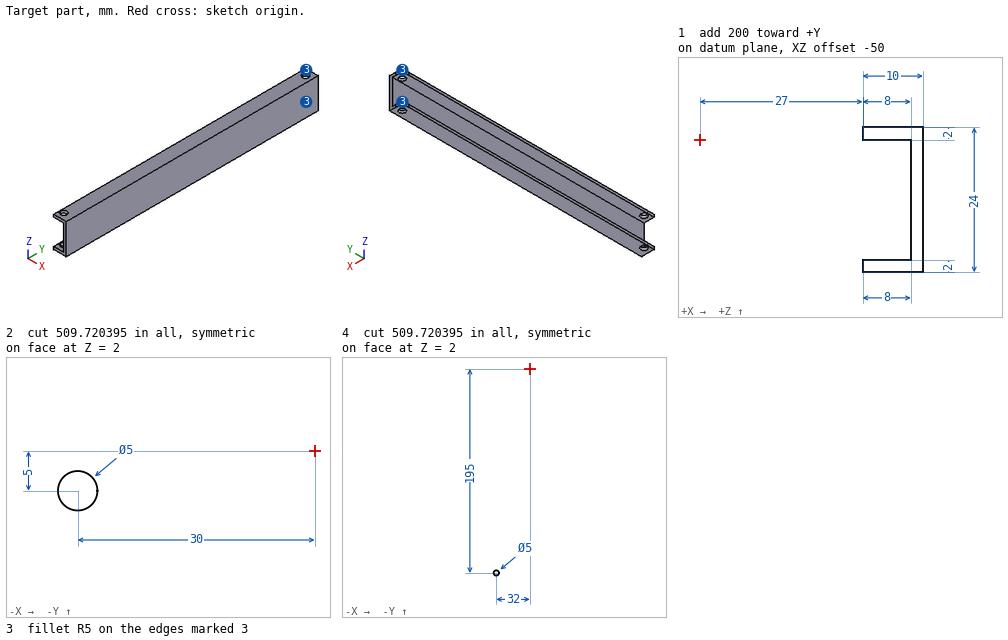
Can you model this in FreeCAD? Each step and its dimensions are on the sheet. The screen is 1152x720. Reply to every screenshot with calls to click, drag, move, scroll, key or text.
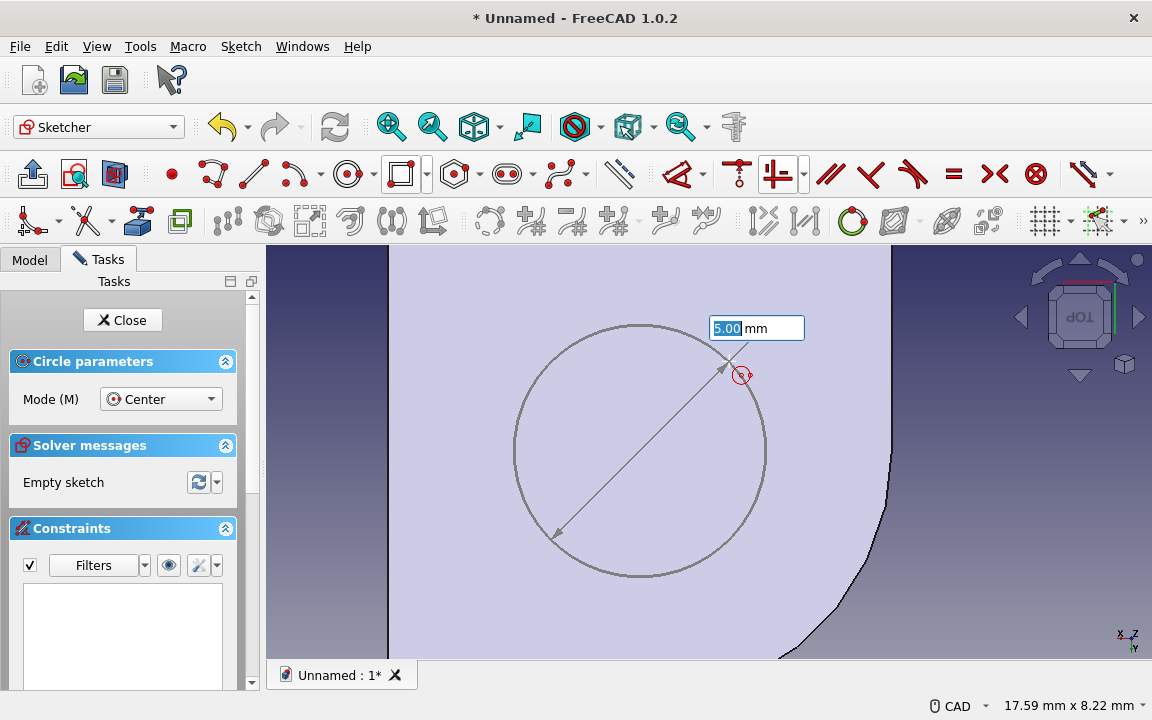
text(5)
key(Return)
key(Escape)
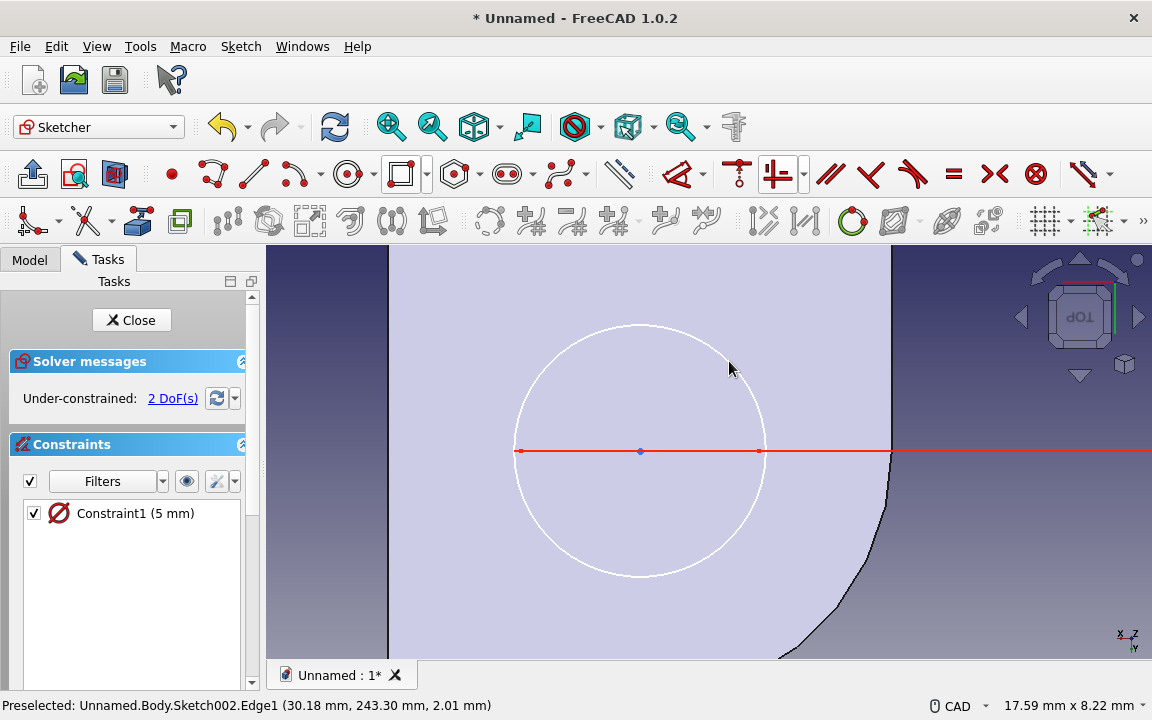
click(676, 174)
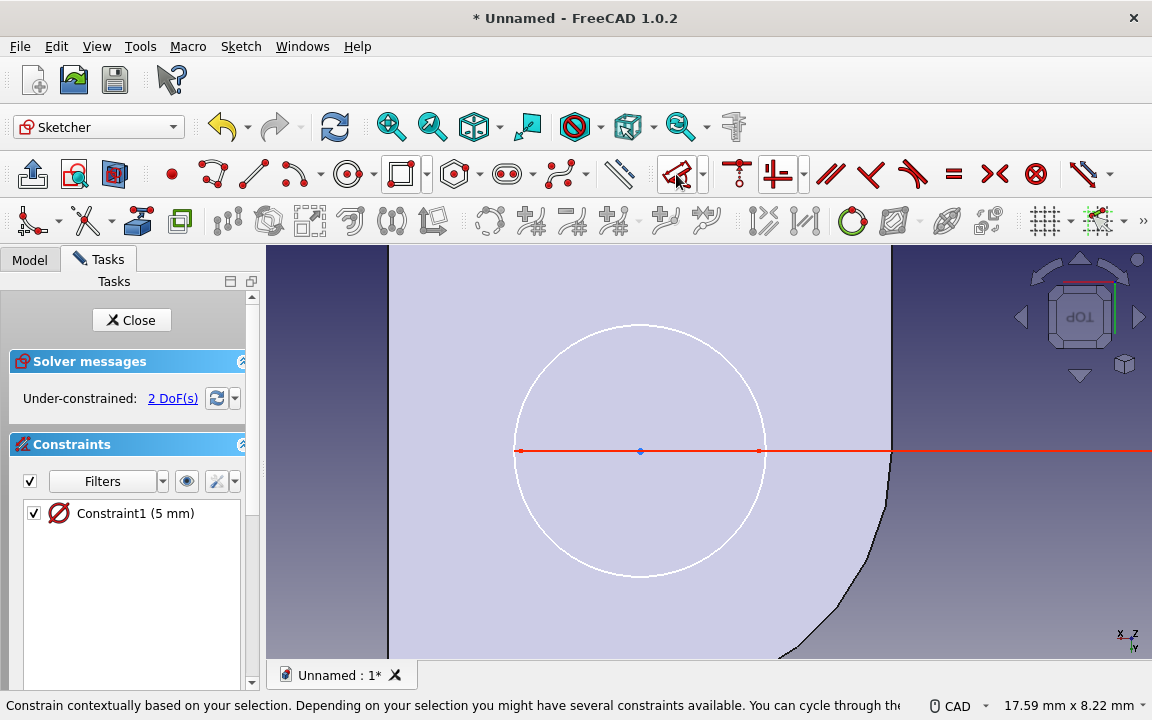
click(640, 451)
click(813, 485)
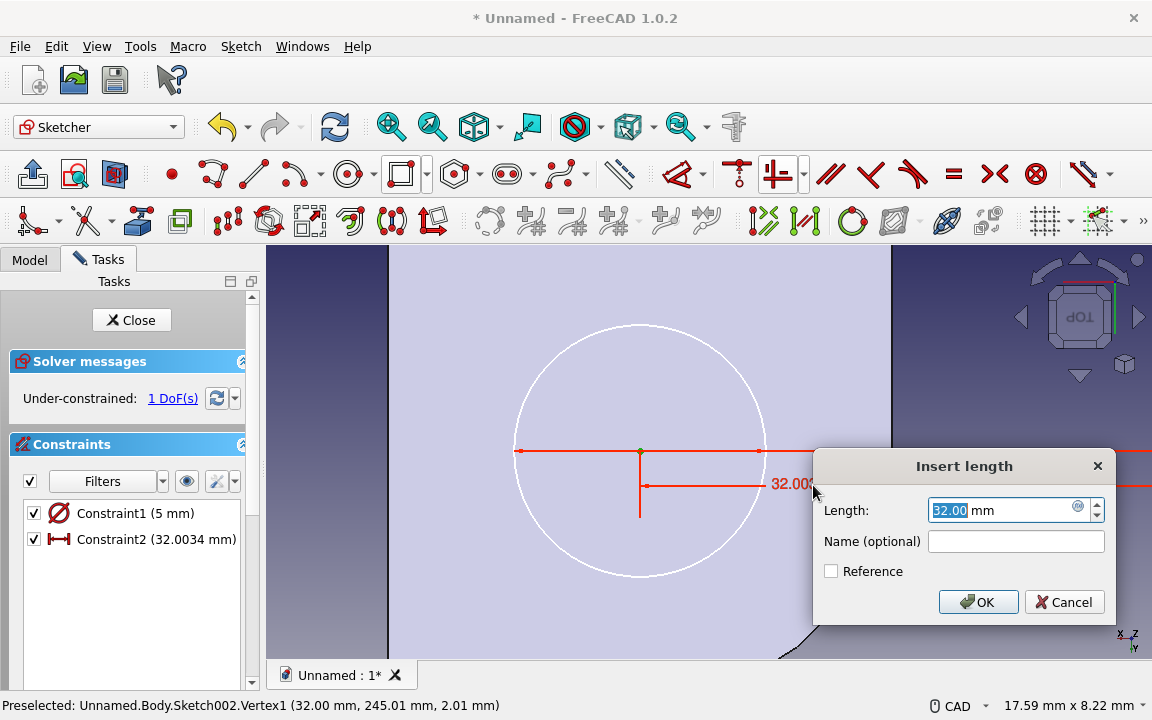
text(32)
key(Return)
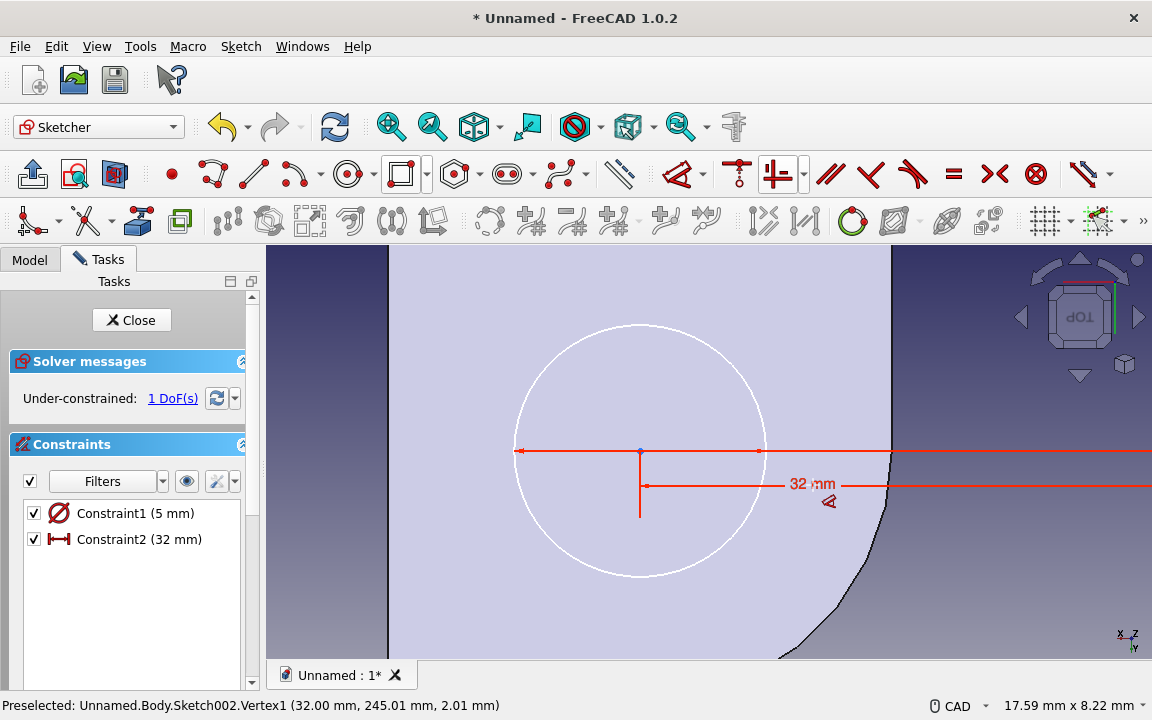
click(640, 451)
click(606, 362)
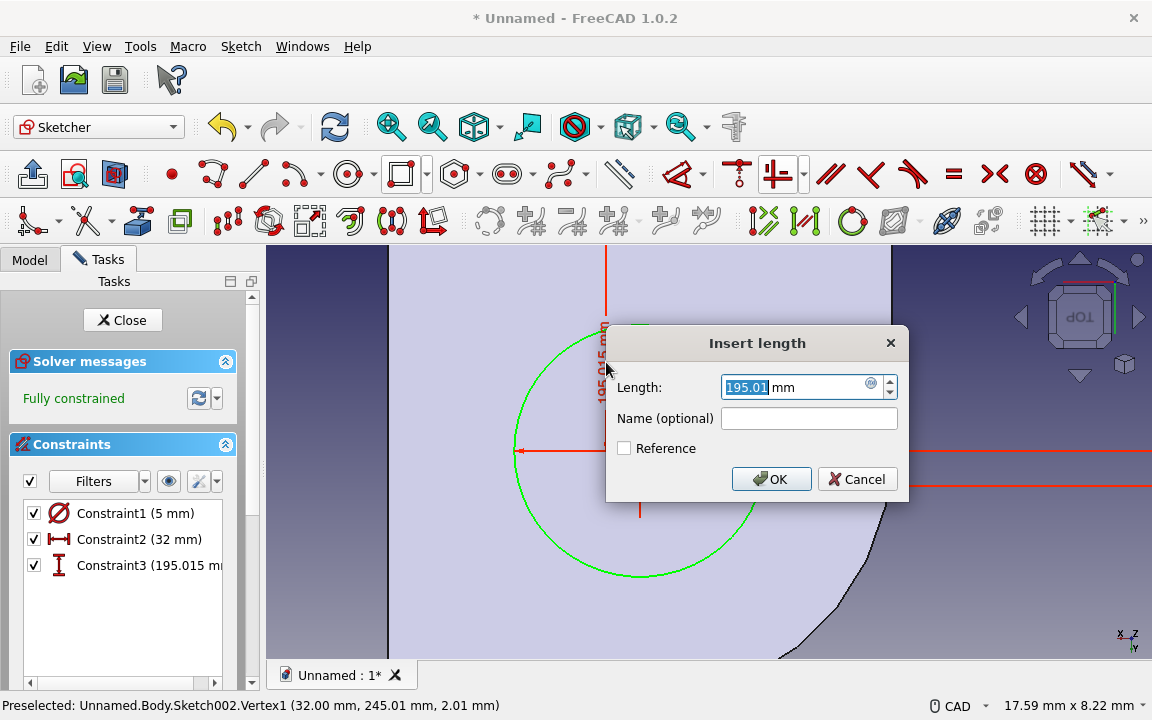
text(195)
key(Return)
key(Escape)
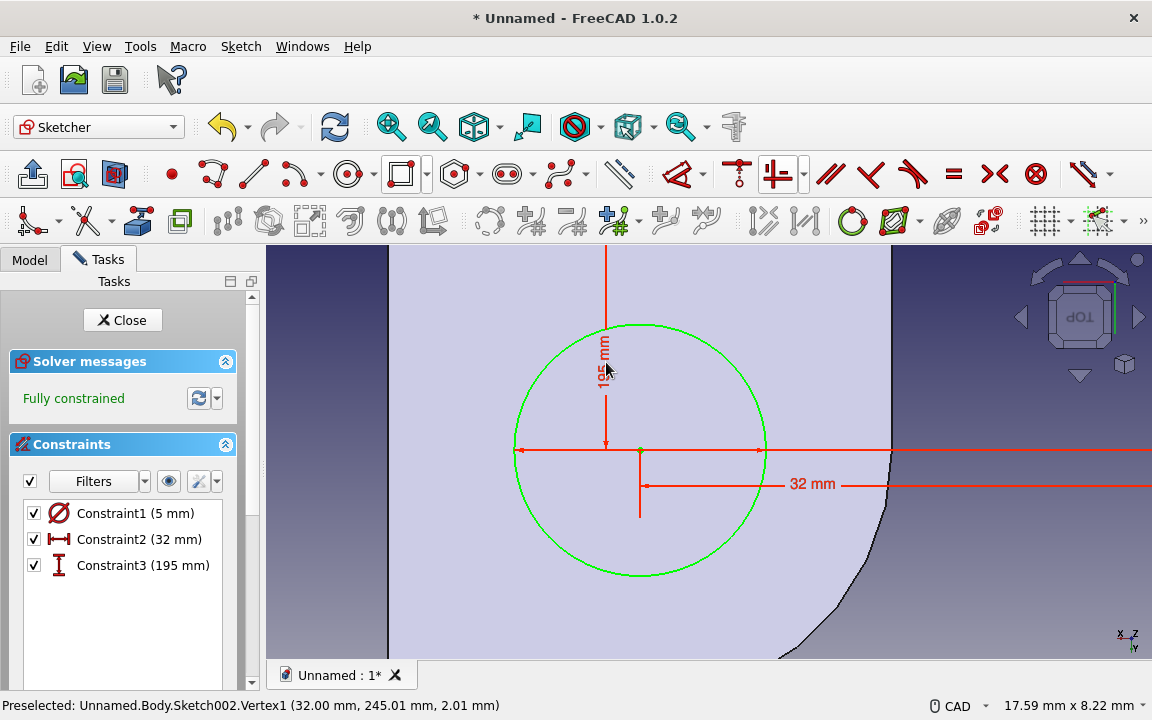
click(123, 320)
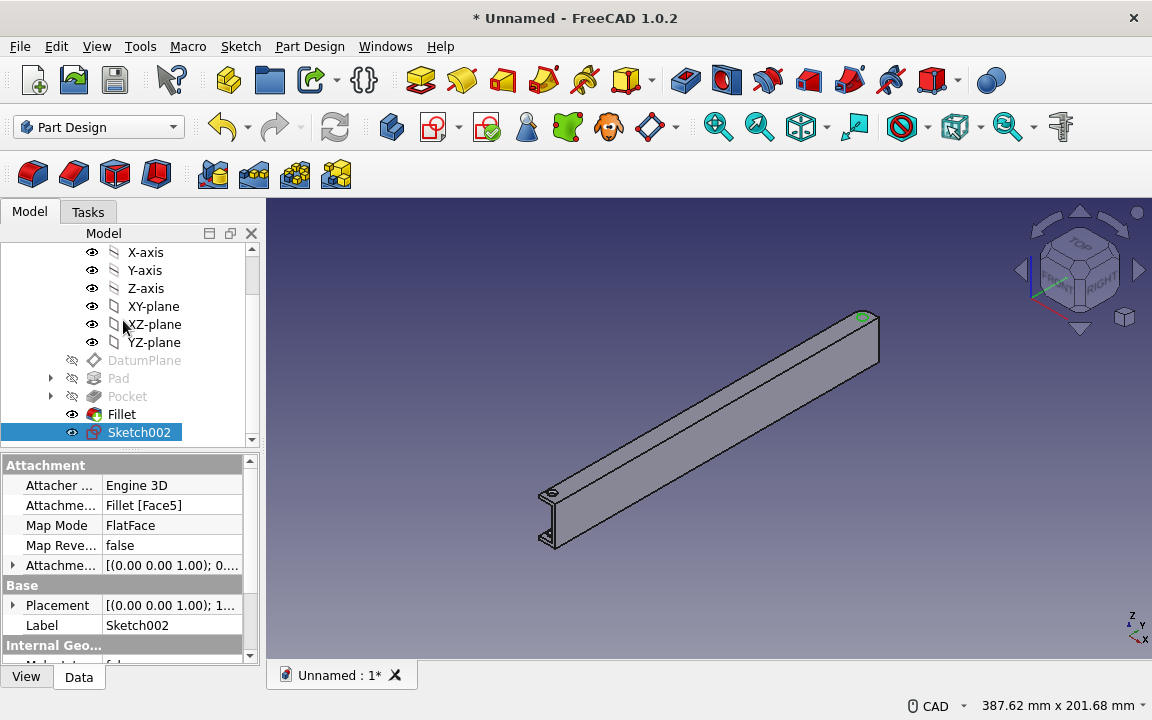
click(686, 80)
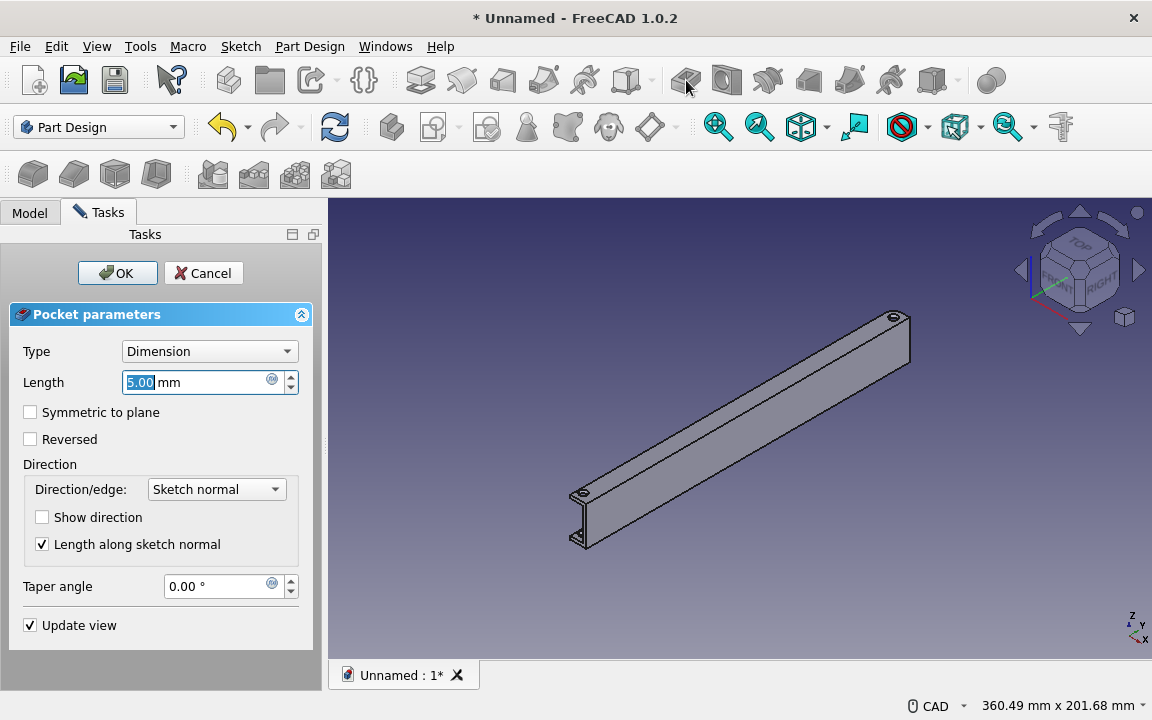
text(509.720395)
key(Tab)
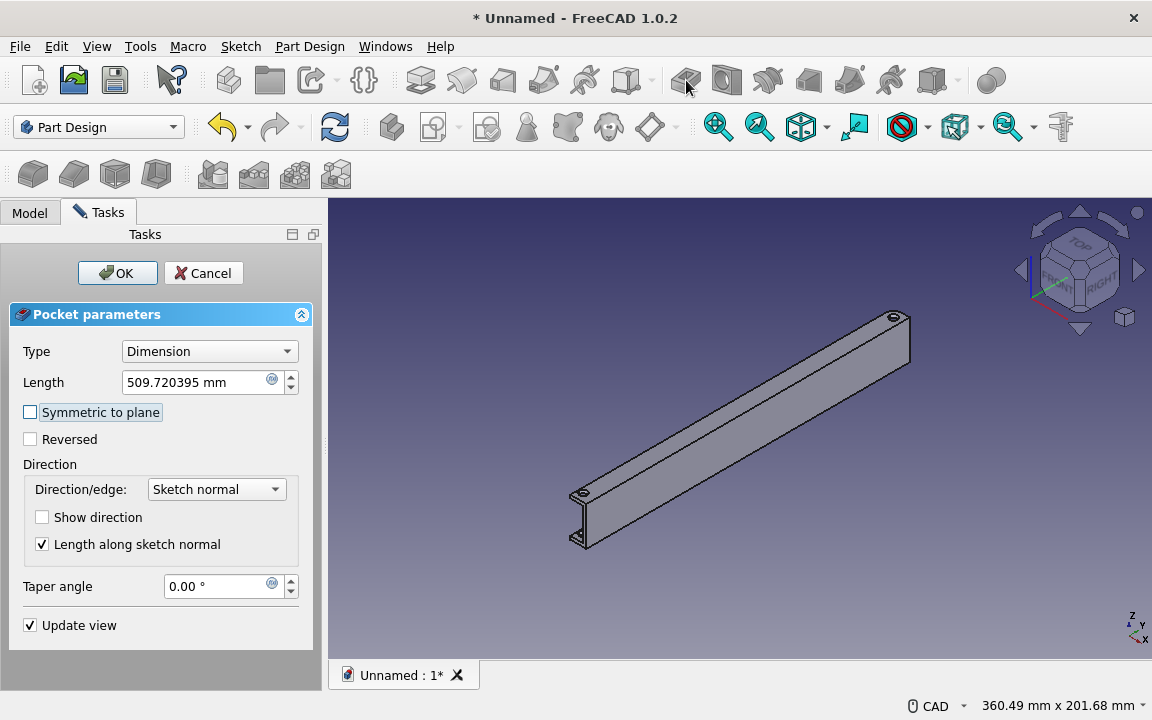
click(31, 412)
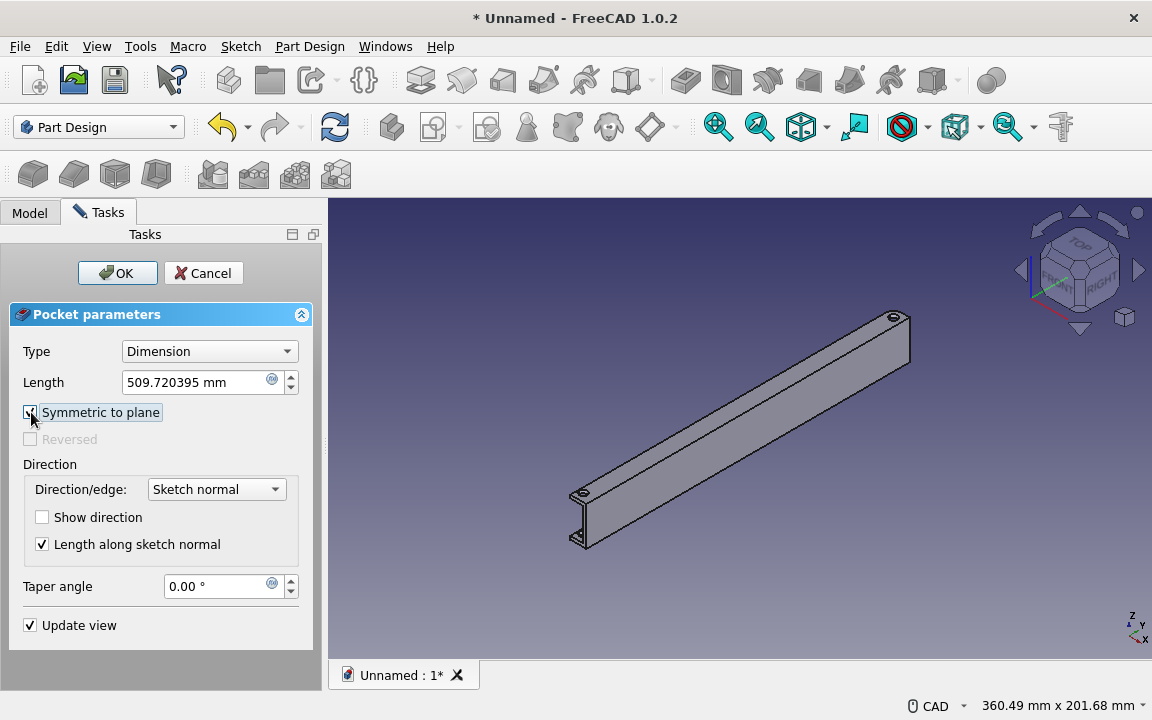
click(118, 273)